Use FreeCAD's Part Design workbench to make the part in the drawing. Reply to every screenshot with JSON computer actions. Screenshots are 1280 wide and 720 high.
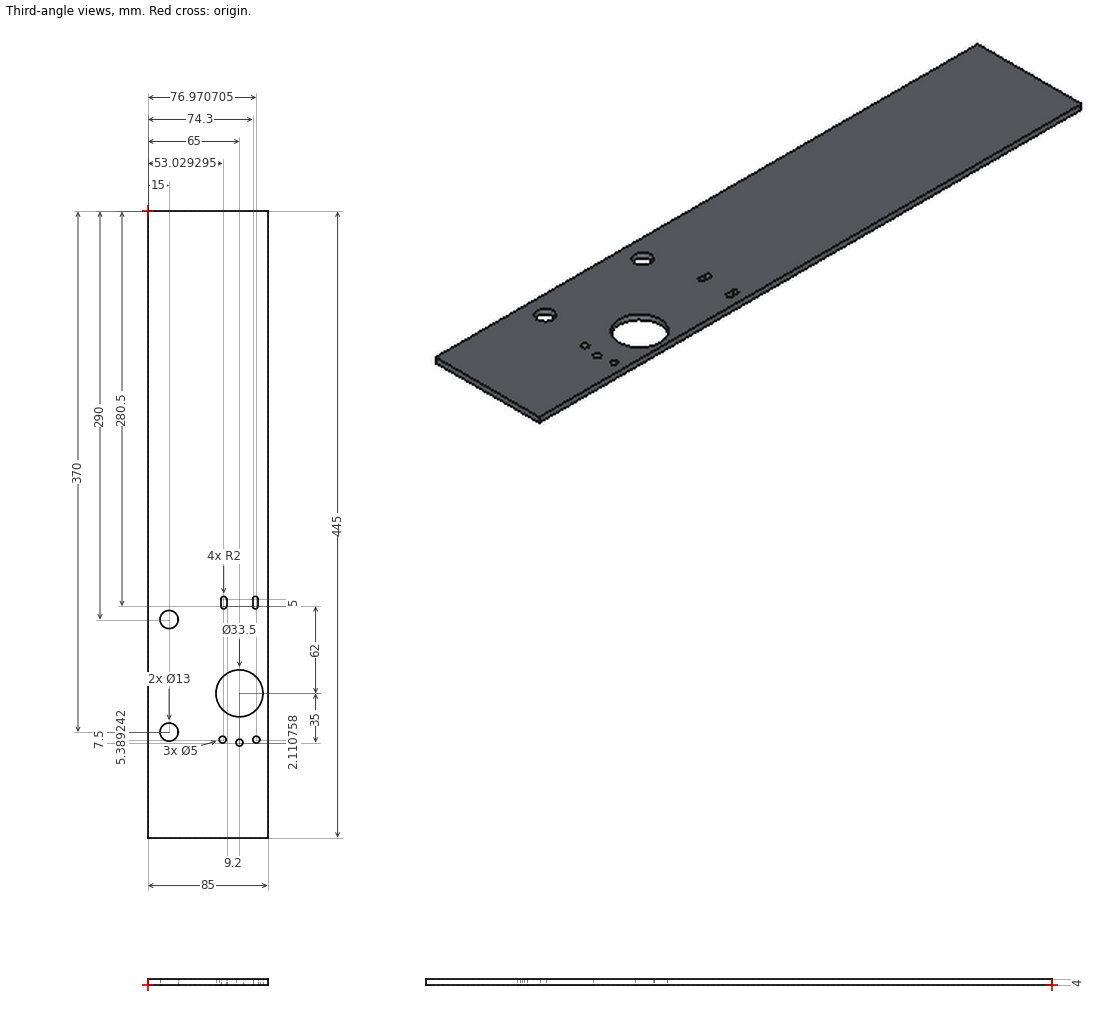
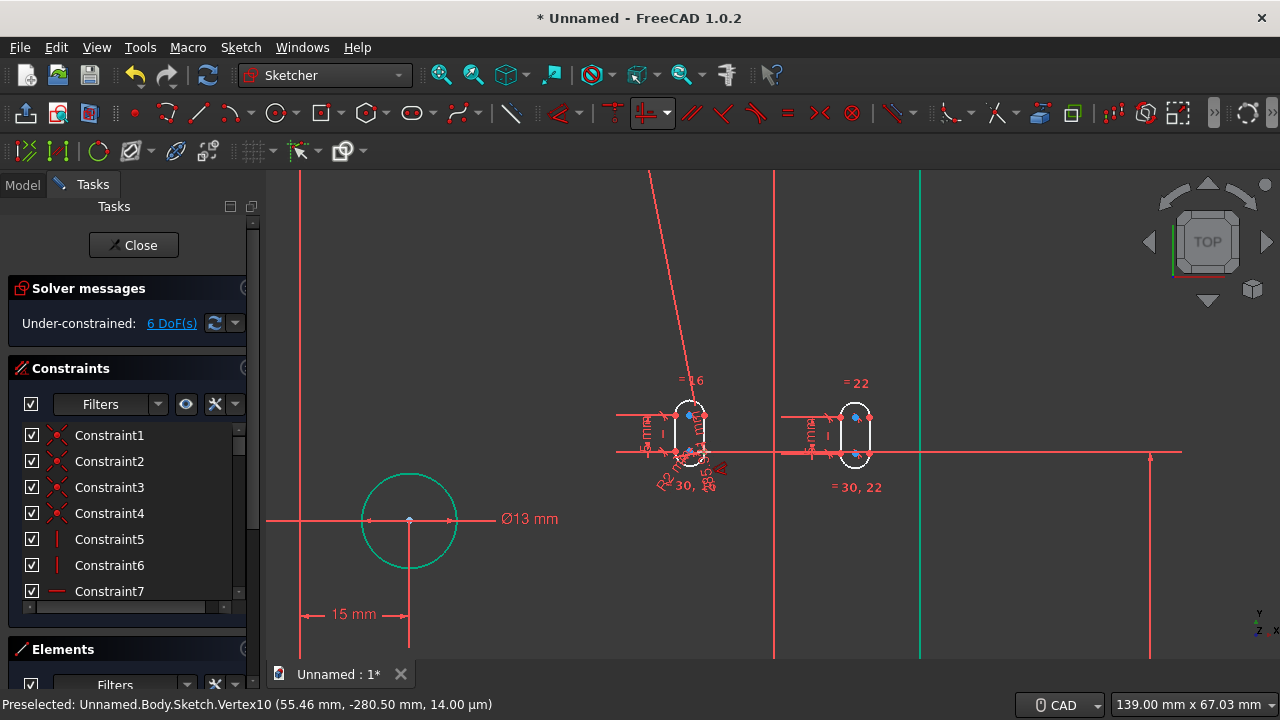
{"action": "scroll", "coordinate": [714, 453], "scroll_direction": "down", "scroll_amount": 12}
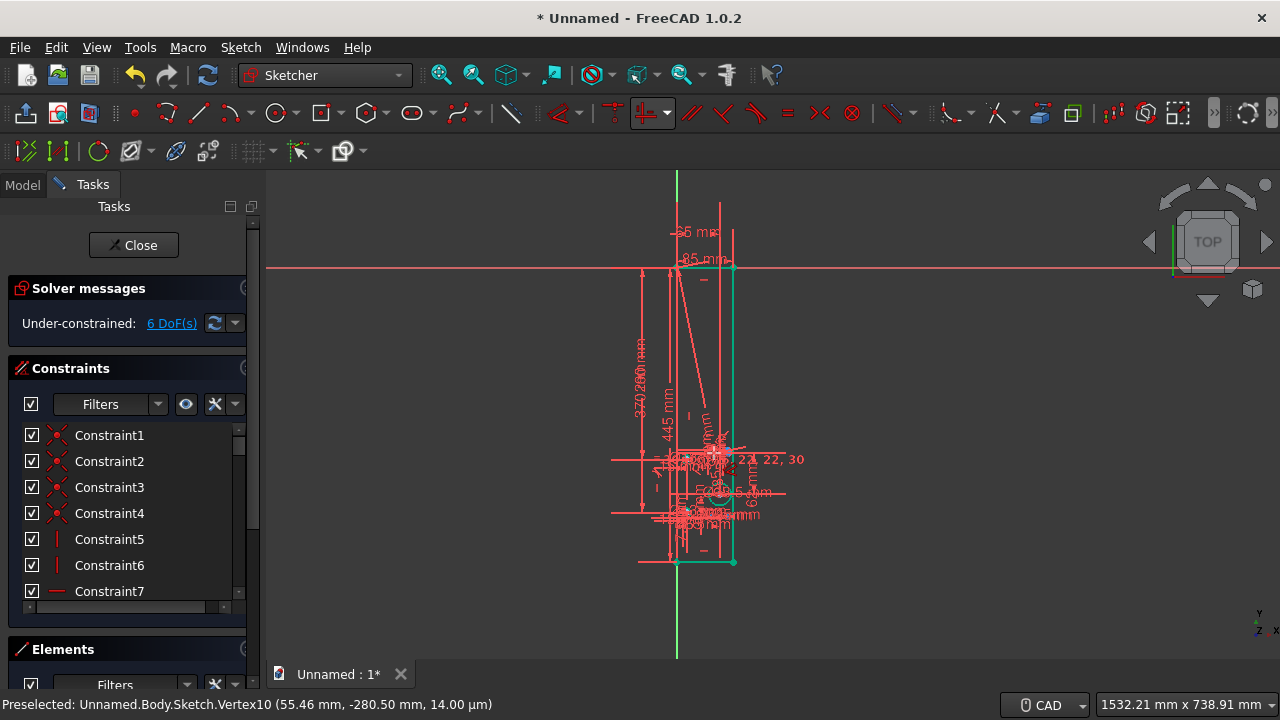
{"action": "scroll", "coordinate": [720, 494], "scroll_direction": "up", "scroll_amount": 10}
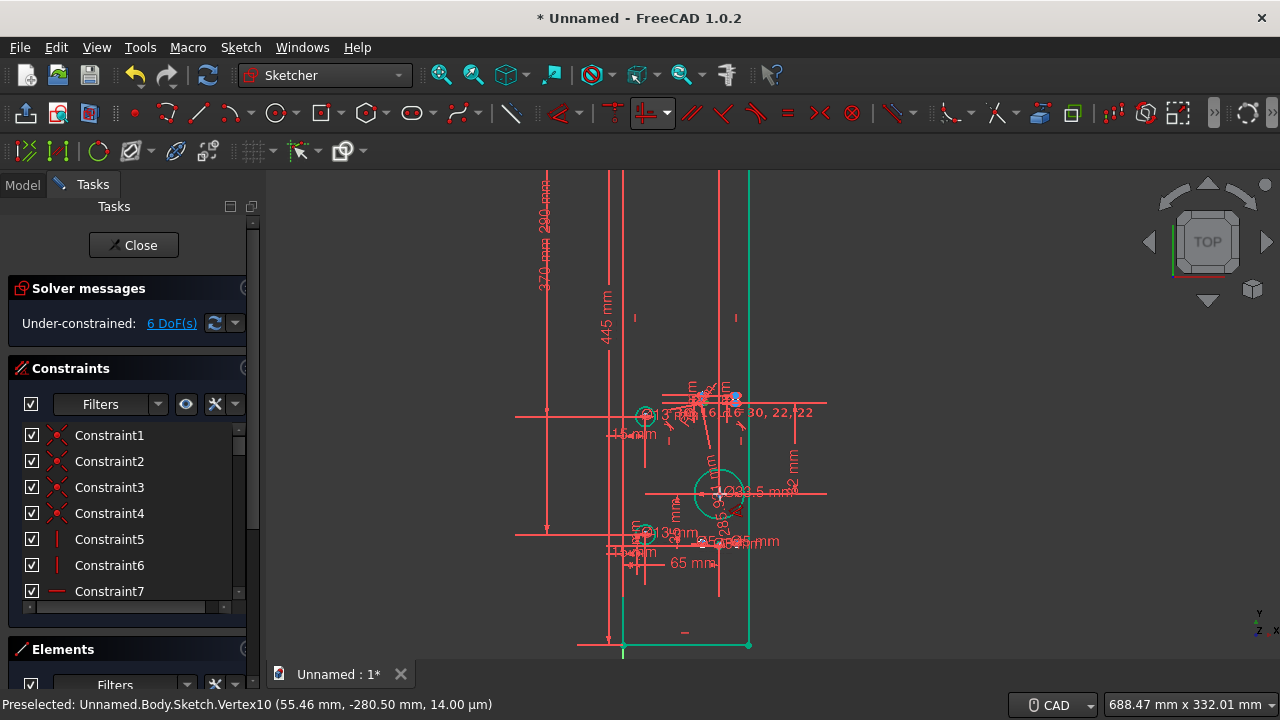
{"action": "left_click", "coordinate": [716, 493]}
{"action": "left_click", "coordinate": [693, 527]}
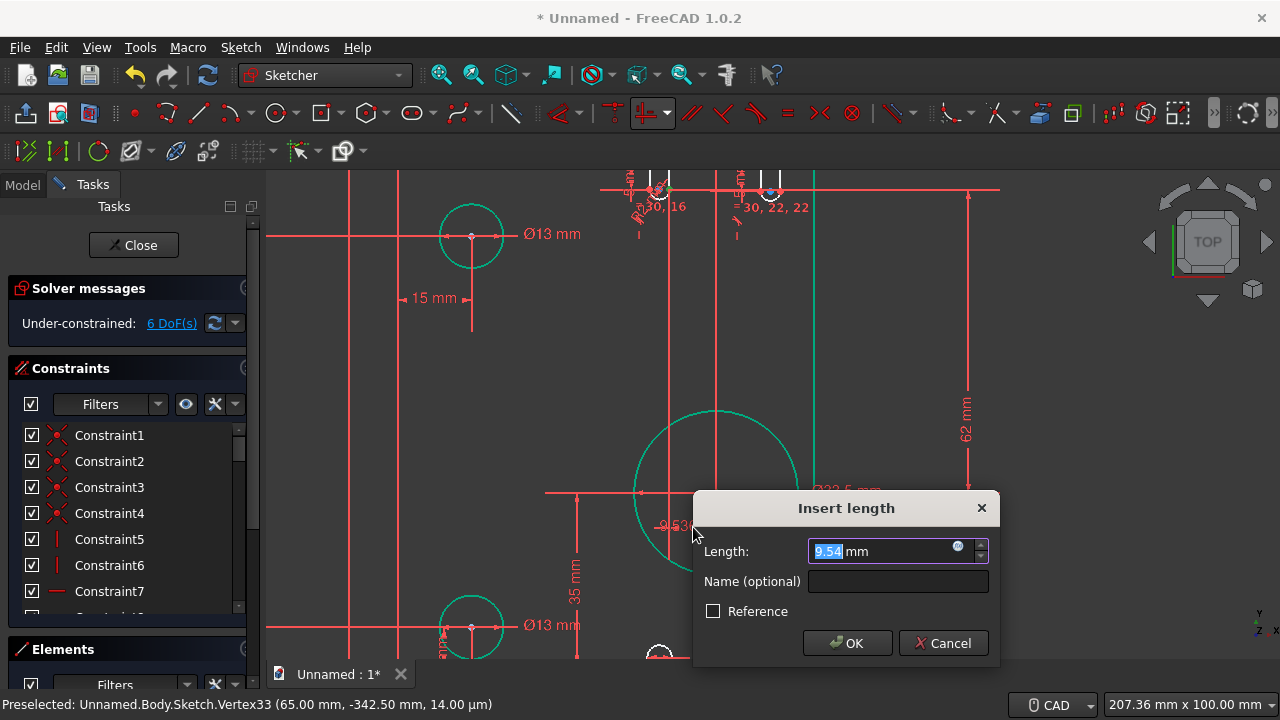
{"action": "type", "text": "9.2"}
{"action": "key", "text": "Return"}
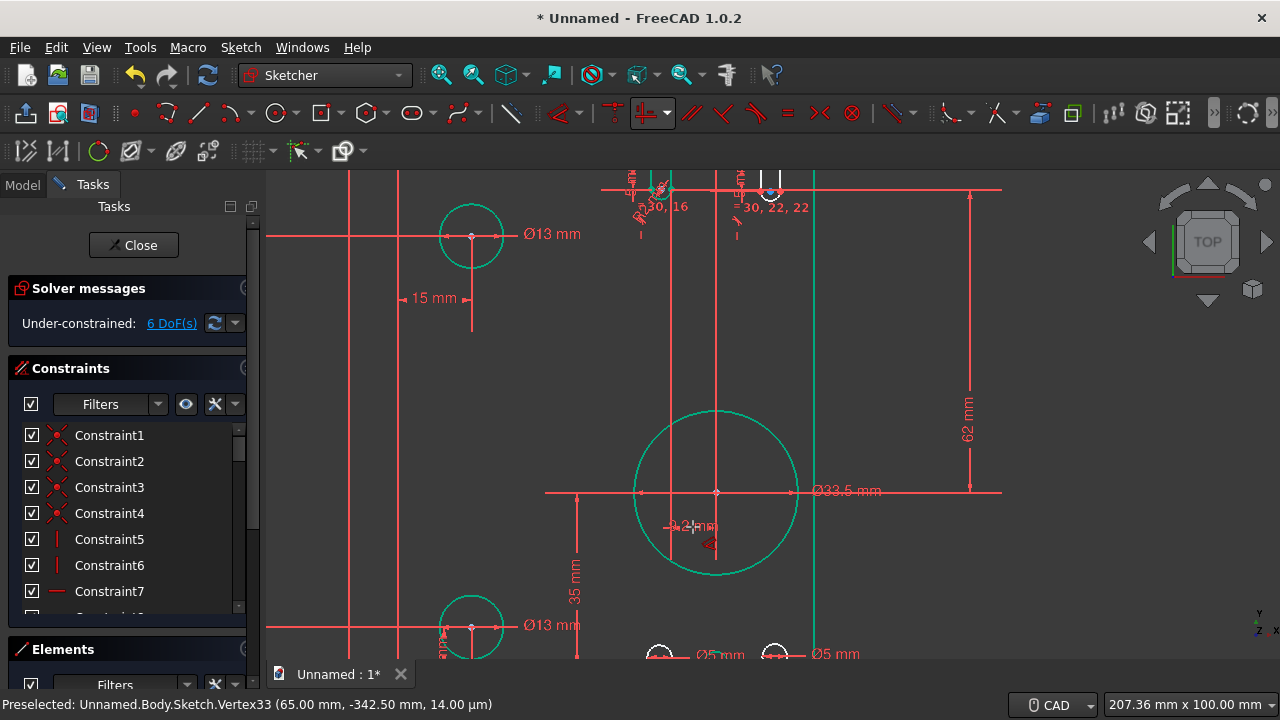
{"action": "scroll", "coordinate": [720, 494], "scroll_direction": "down", "scroll_amount": 10}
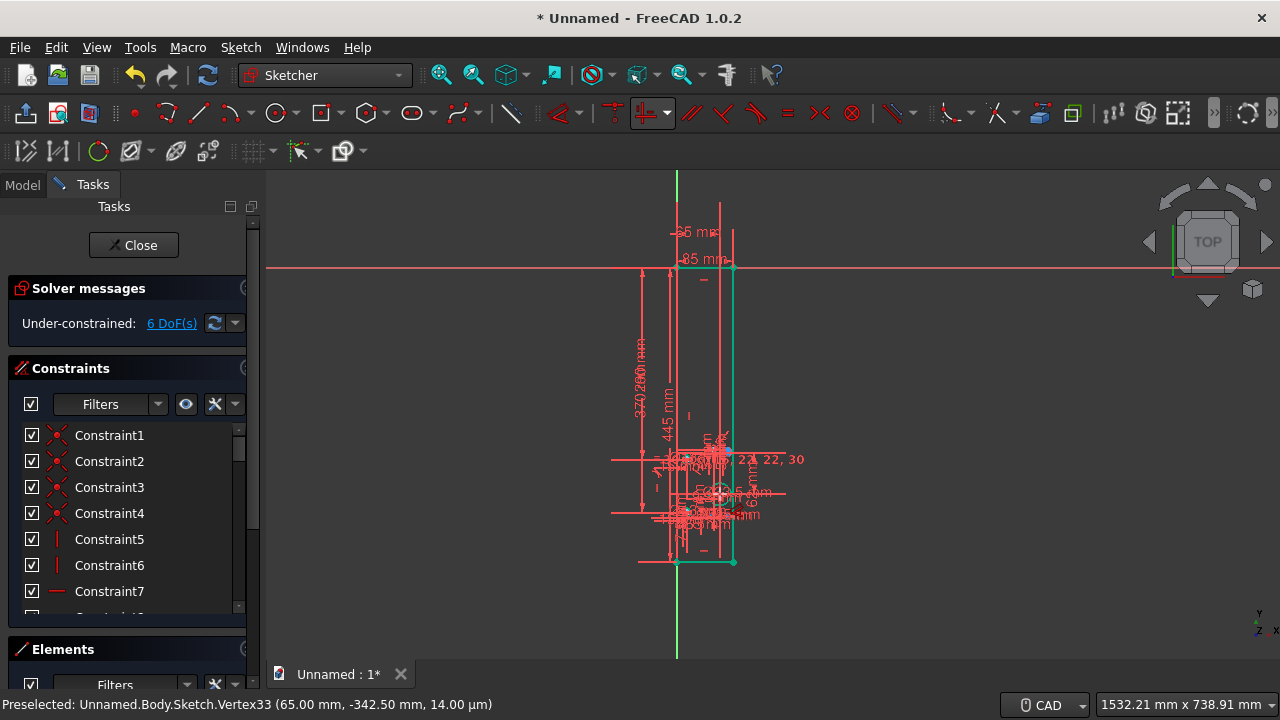
{"action": "scroll", "coordinate": [726, 454], "scroll_direction": "up", "scroll_amount": 12}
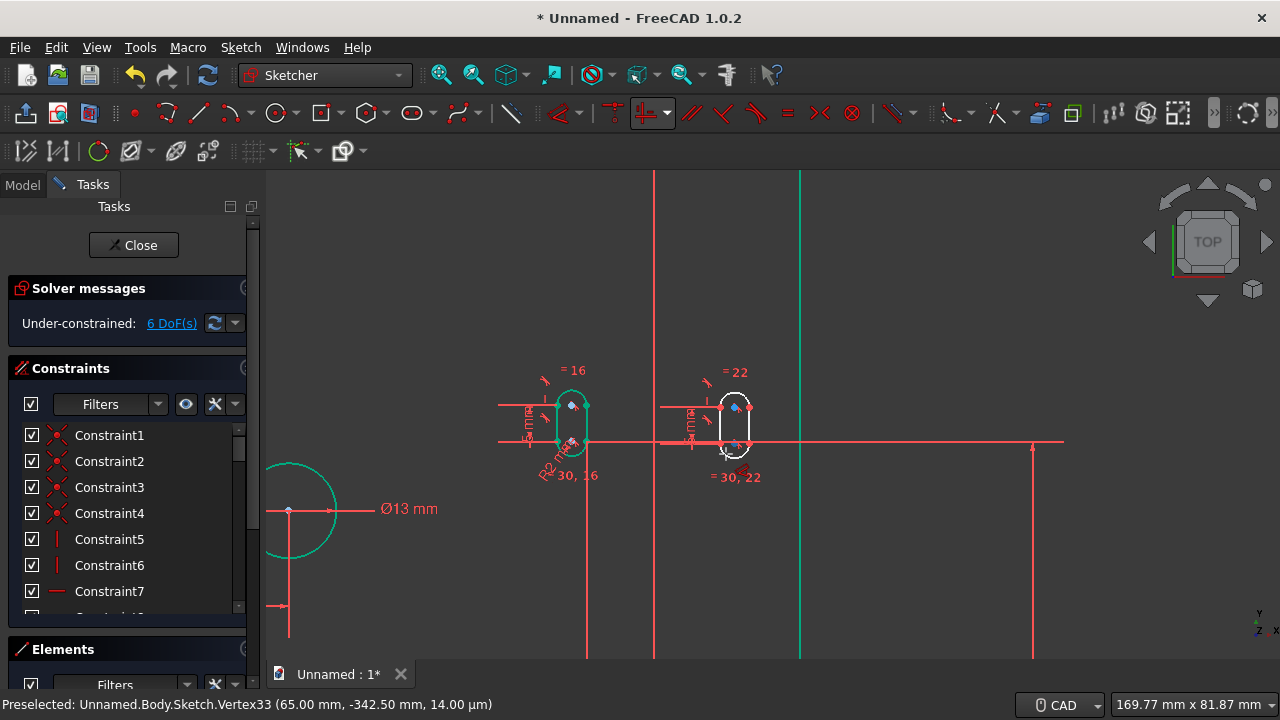
{"action": "left_click", "coordinate": [720, 444]}
{"action": "left_click", "coordinate": [409, 478]}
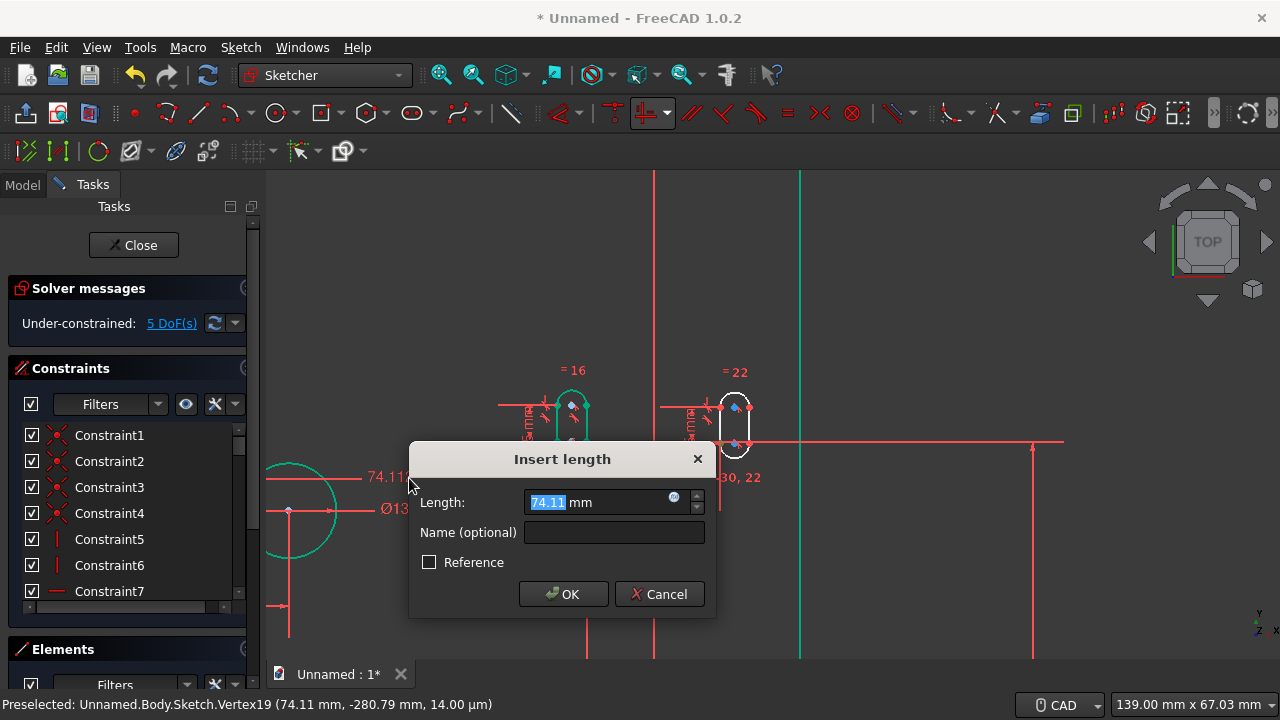
{"action": "type", "text": "74.3"}
{"action": "key", "text": "Return"}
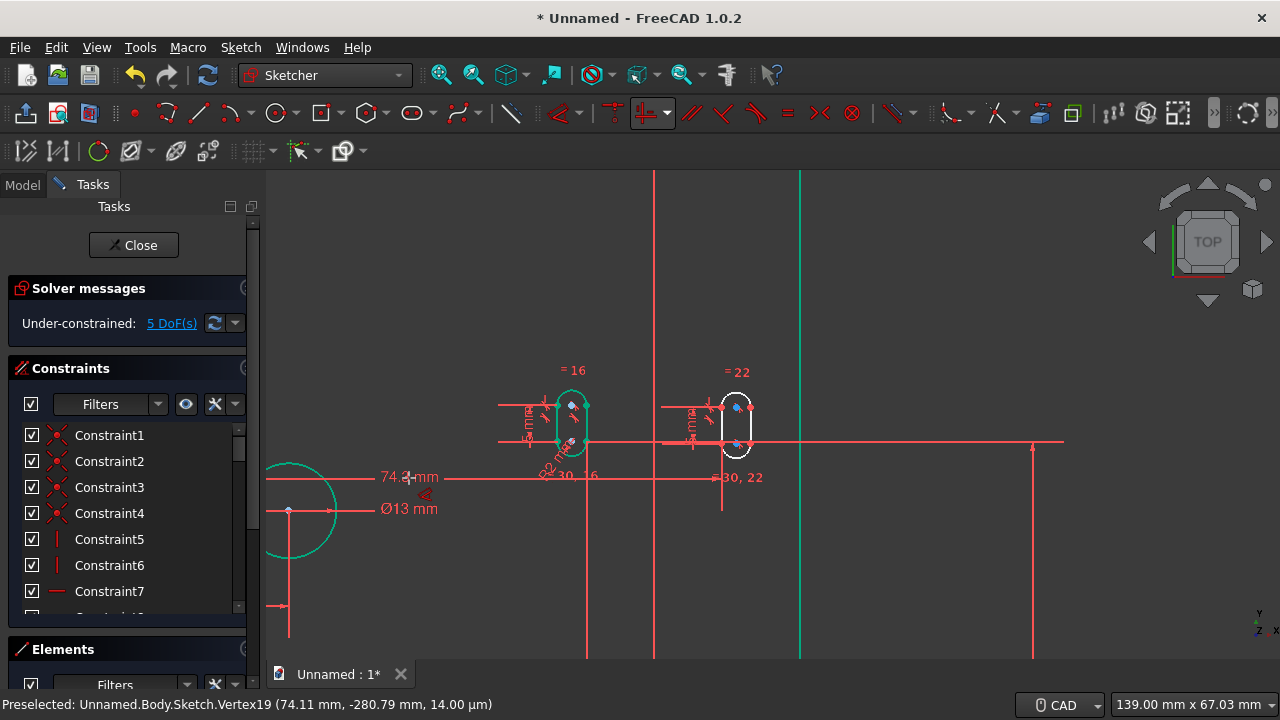
{"action": "left_click", "coordinate": [722, 444]}
{"action": "left_click", "coordinate": [756, 321]}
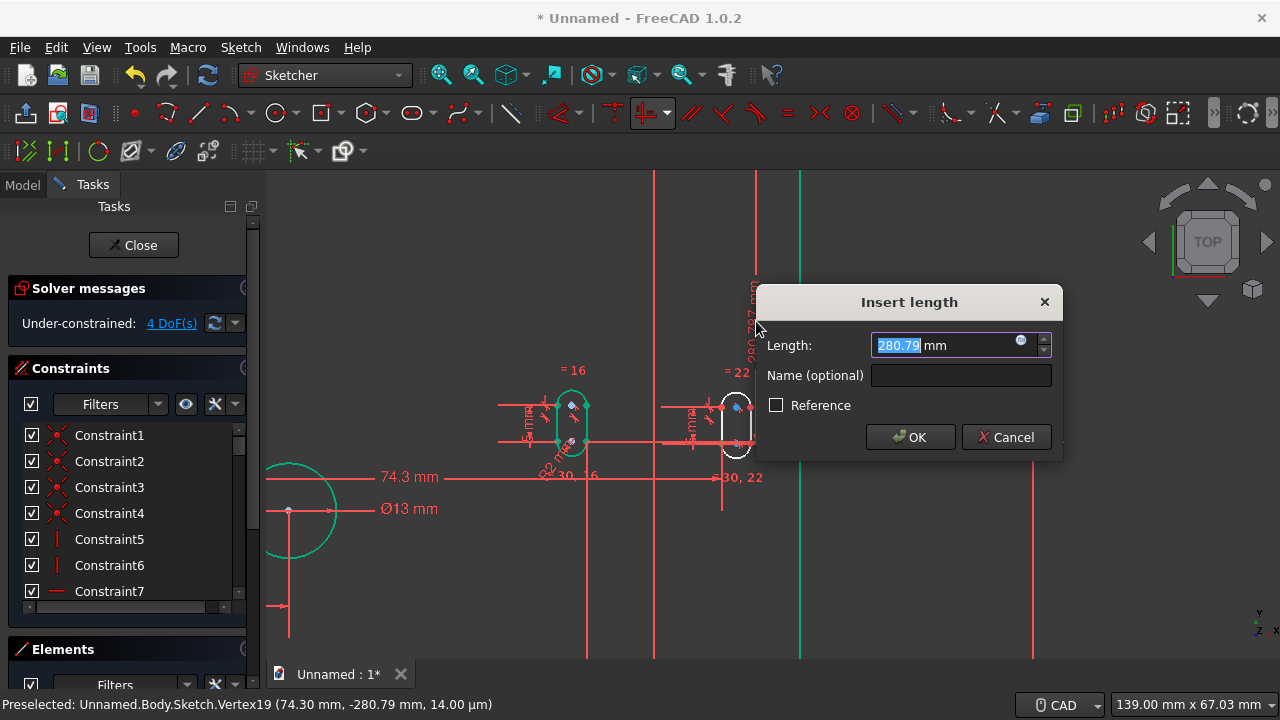
{"action": "type", "text": "280.5"}
{"action": "key", "text": "Return"}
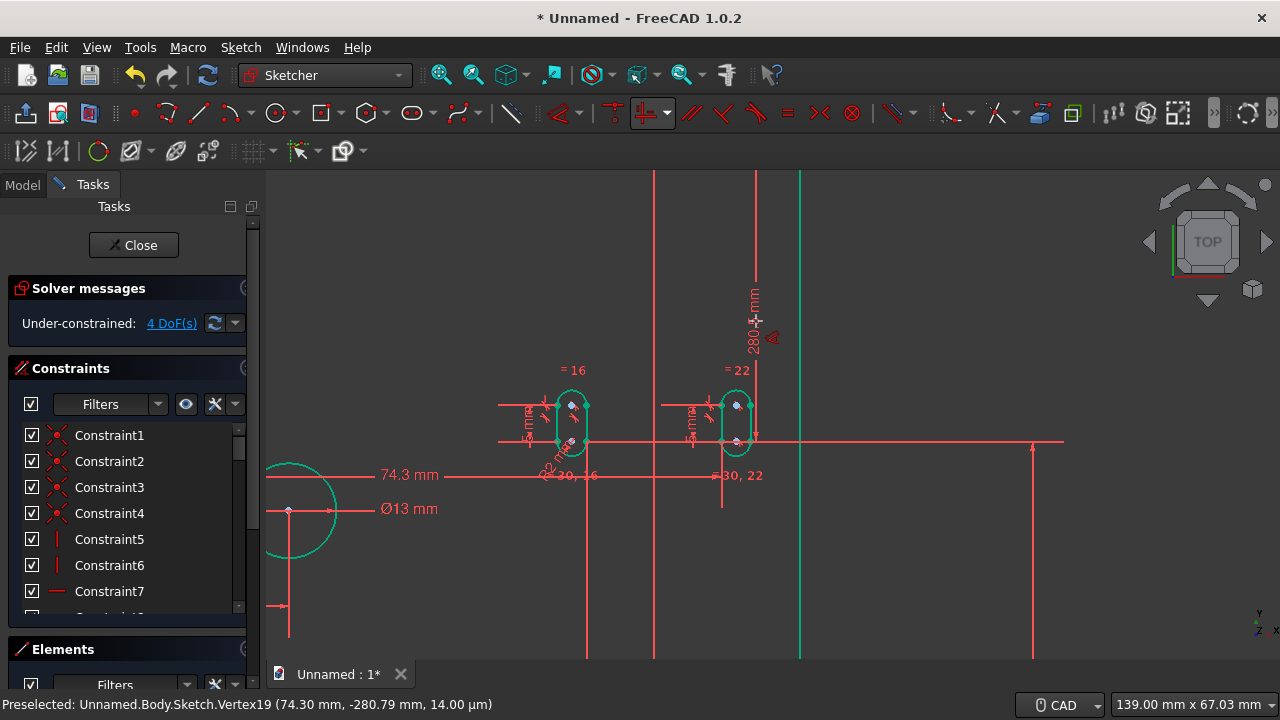
{"action": "scroll", "coordinate": [726, 454], "scroll_direction": "down", "scroll_amount": 12}